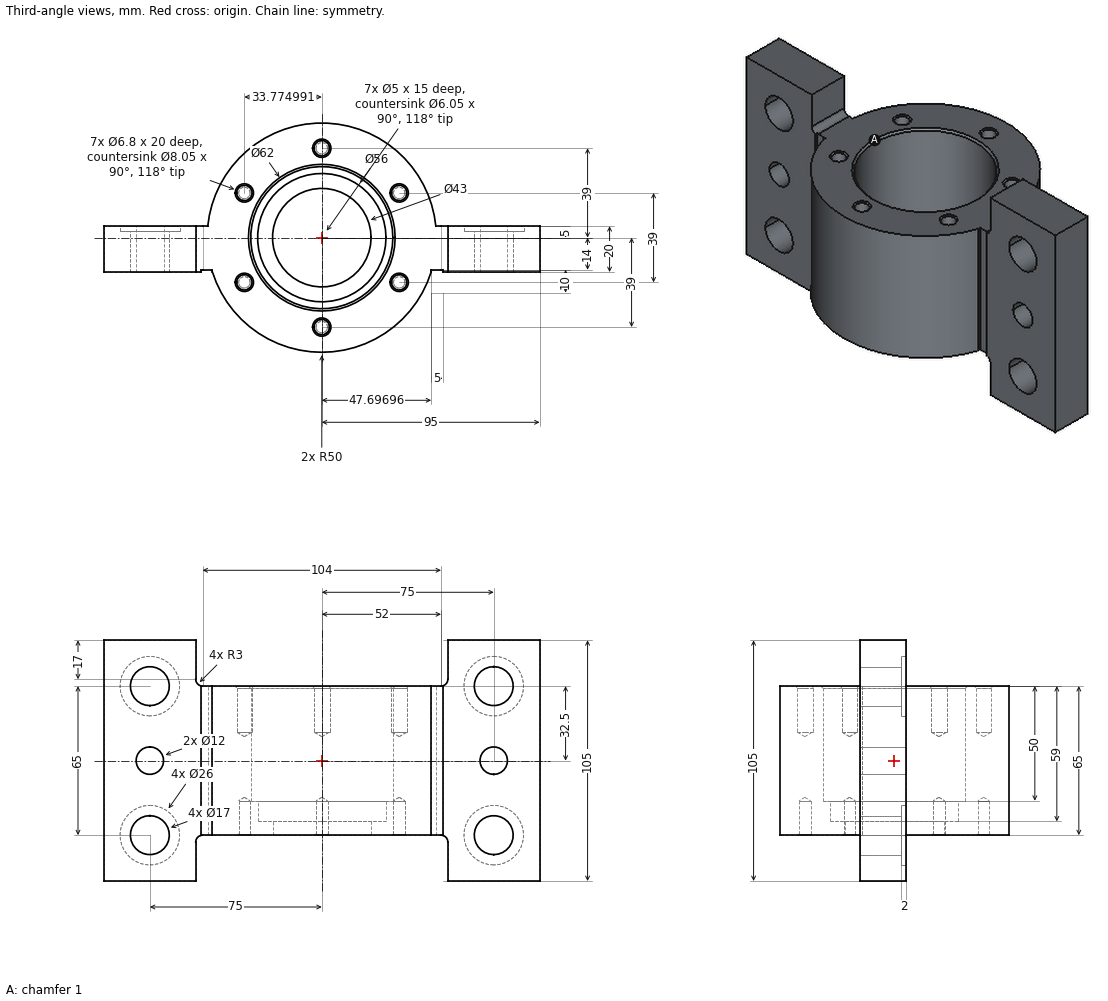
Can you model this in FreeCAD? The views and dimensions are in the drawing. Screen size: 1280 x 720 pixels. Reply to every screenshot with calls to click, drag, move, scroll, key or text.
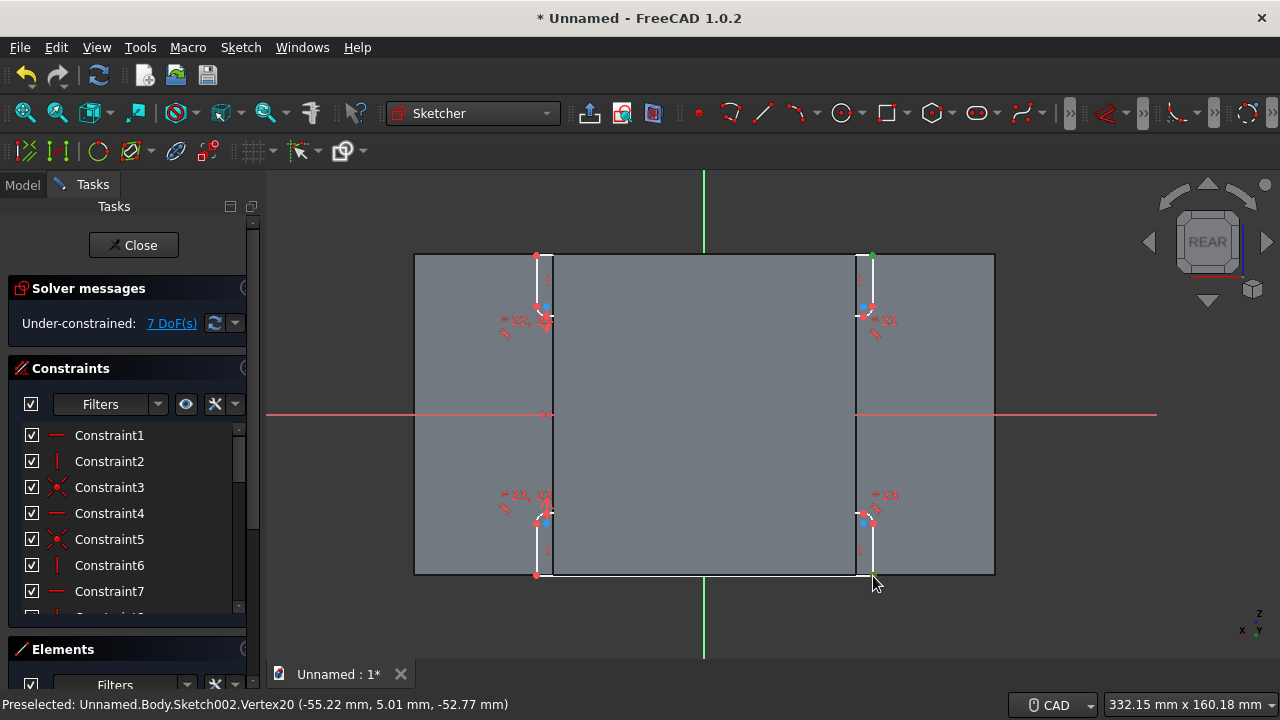
click(353, 415)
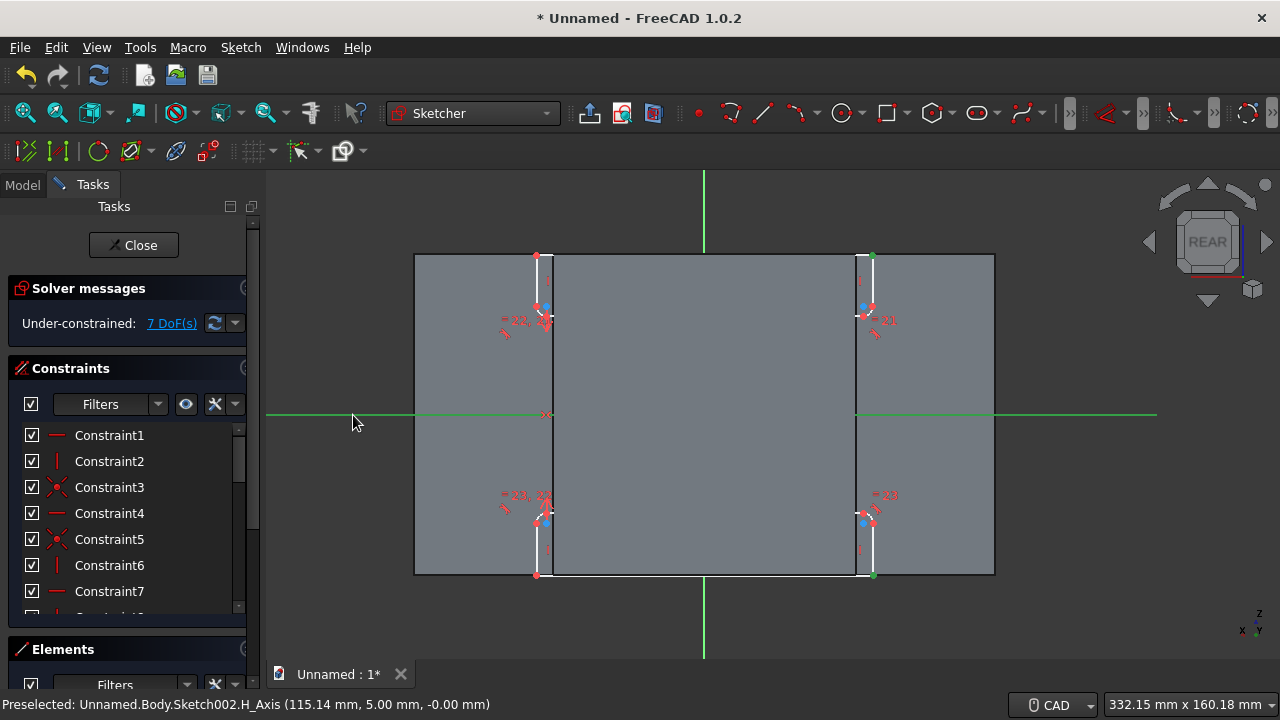
key(s)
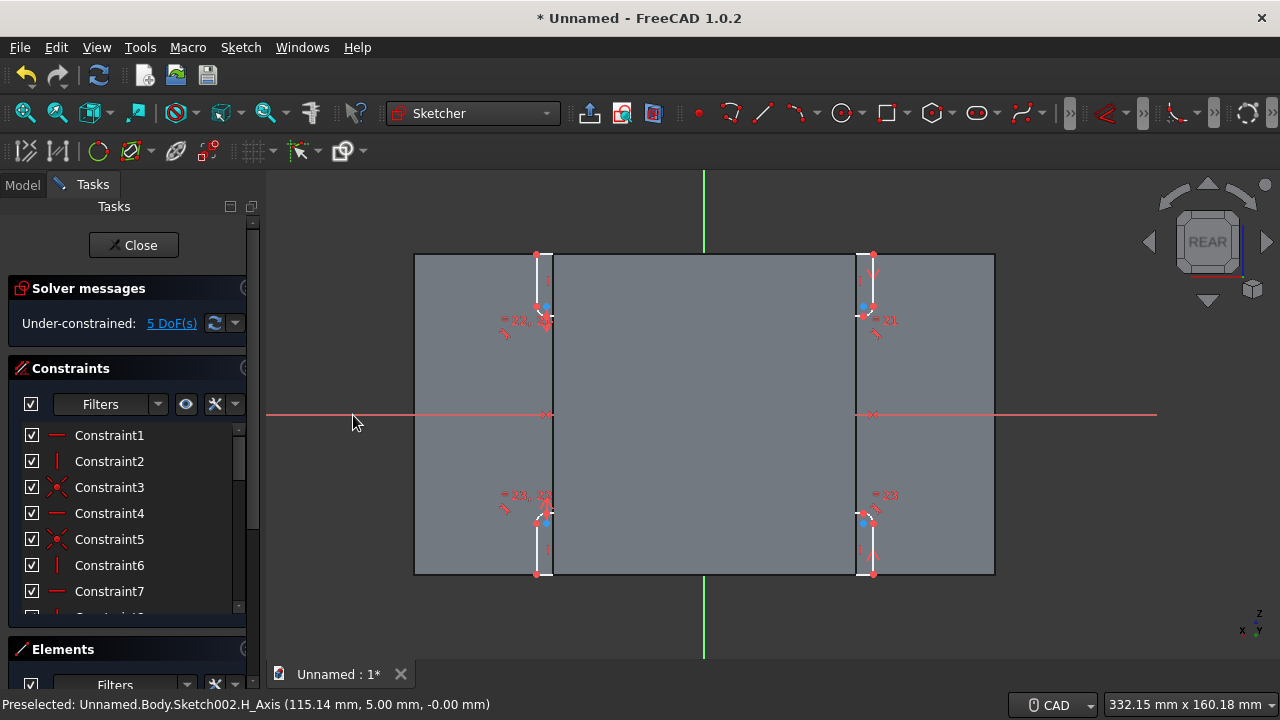
click(1106, 114)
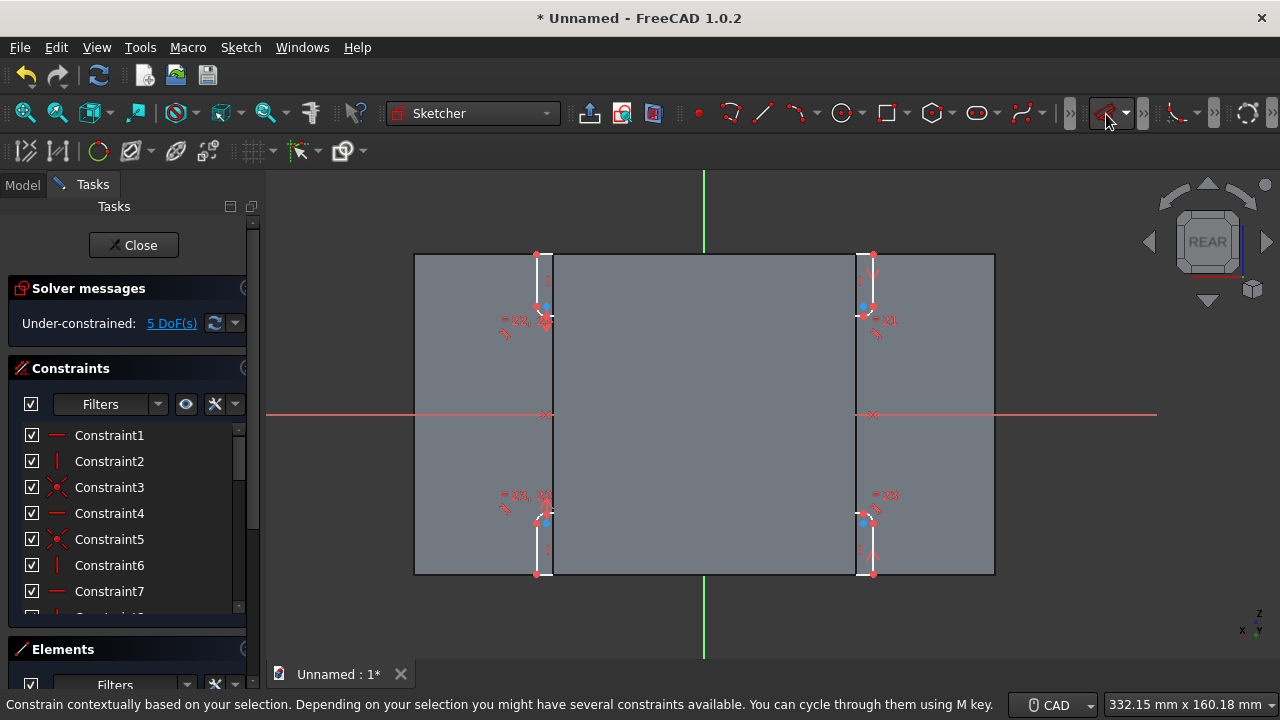
scroll(870, 313, up, 8)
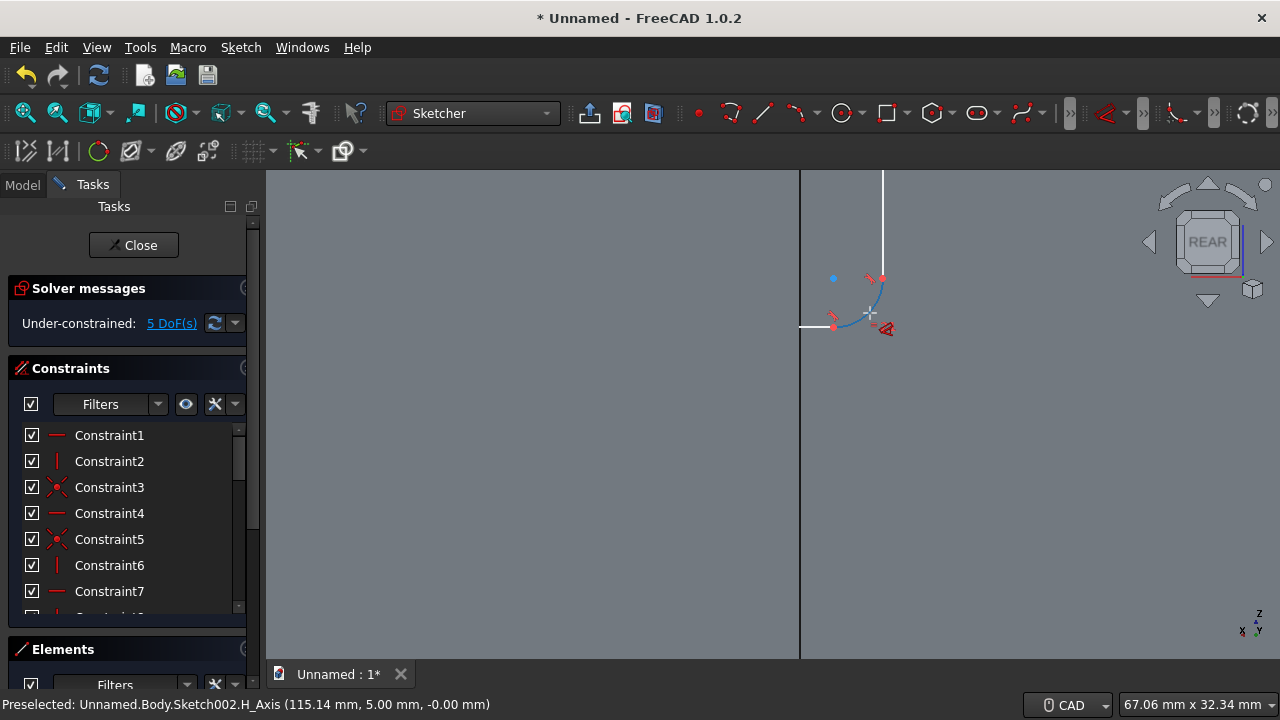
click(869, 313)
click(892, 335)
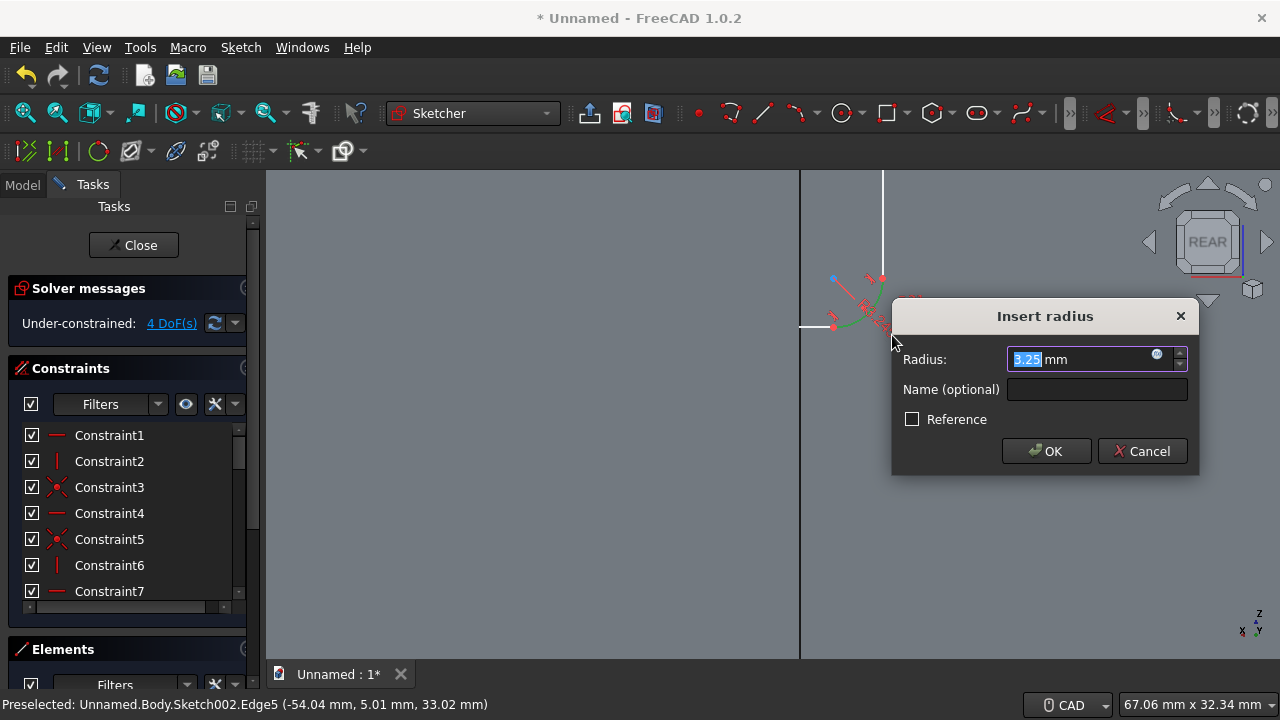
text(3)
key(Return)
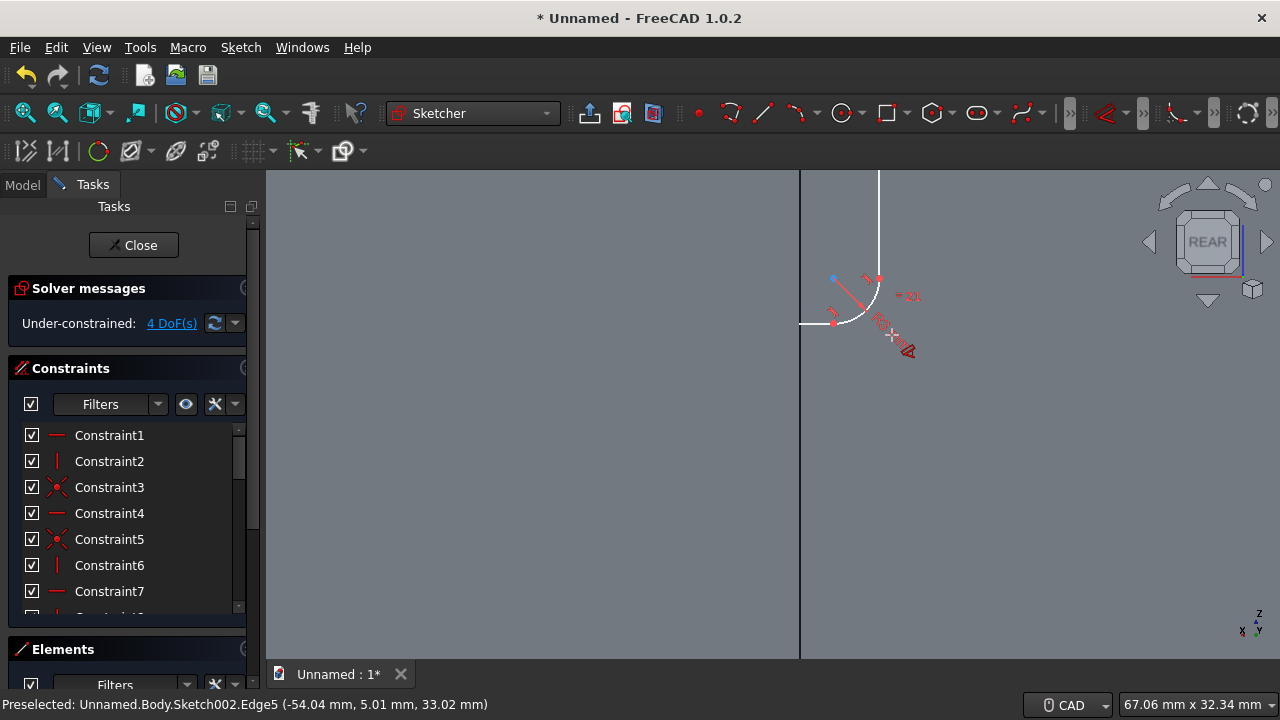
scroll(871, 313, down, 8)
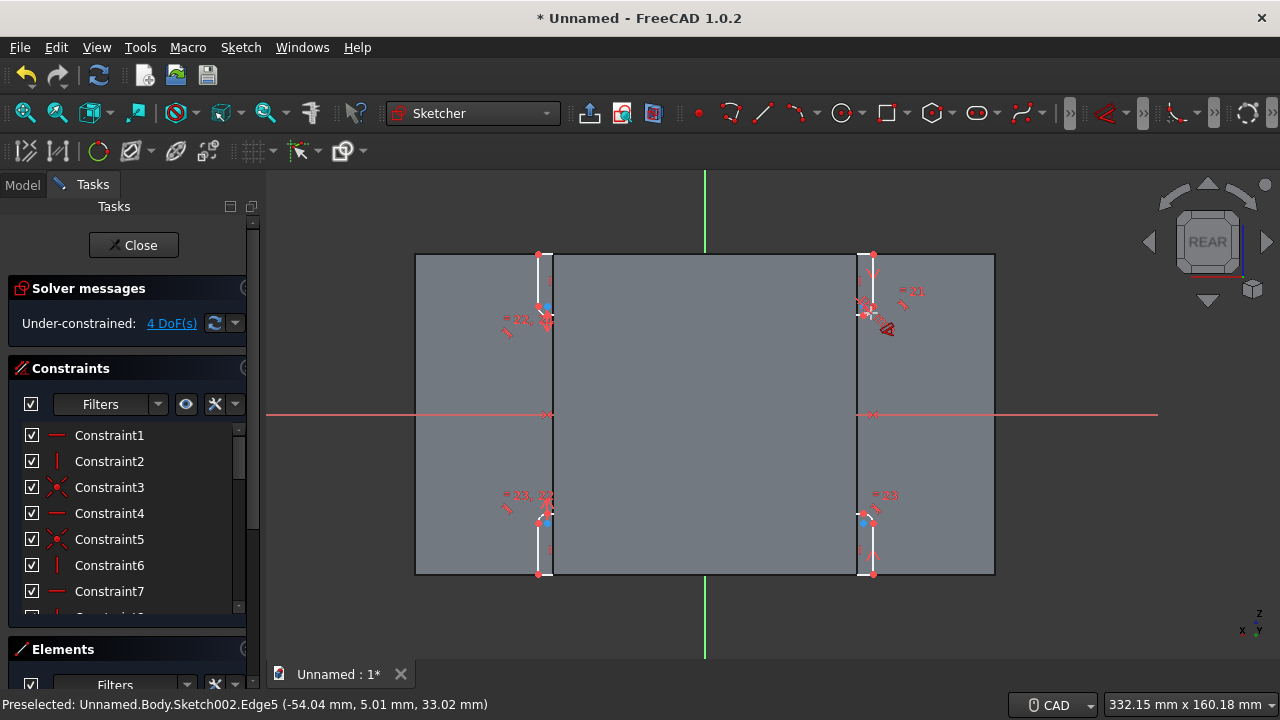
click(873, 291)
click(907, 280)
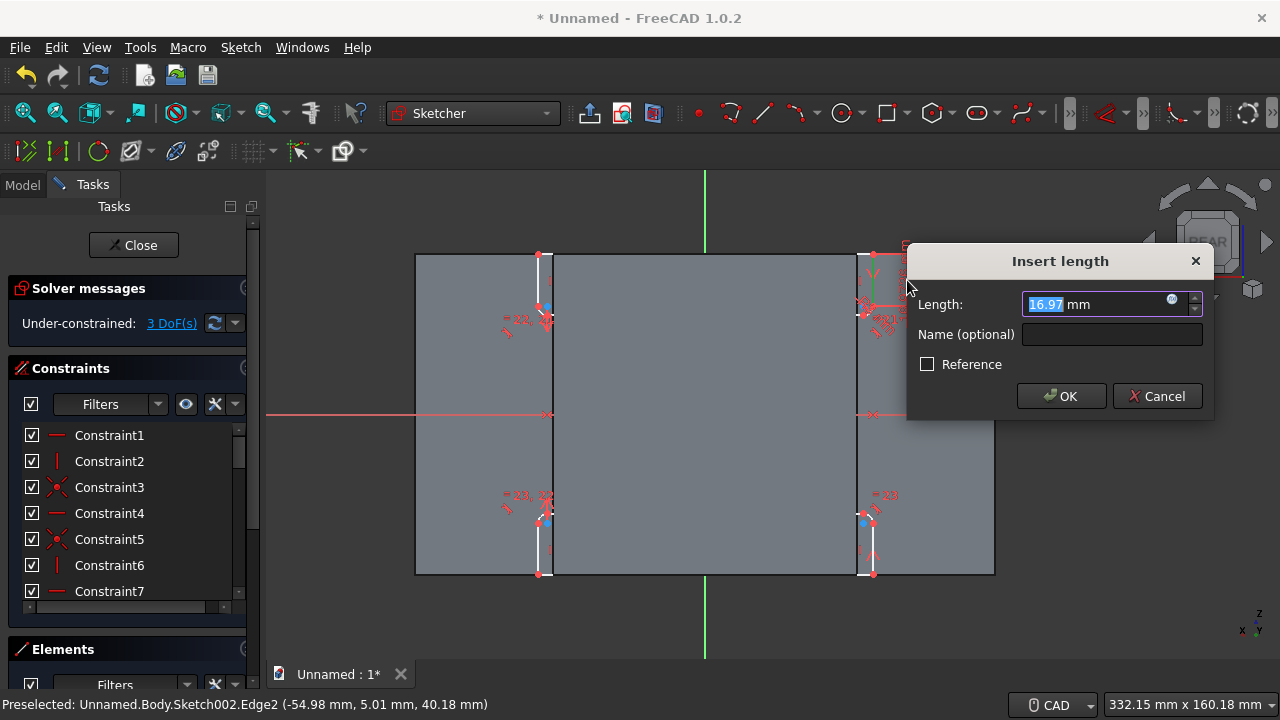
text(17)
key(Return)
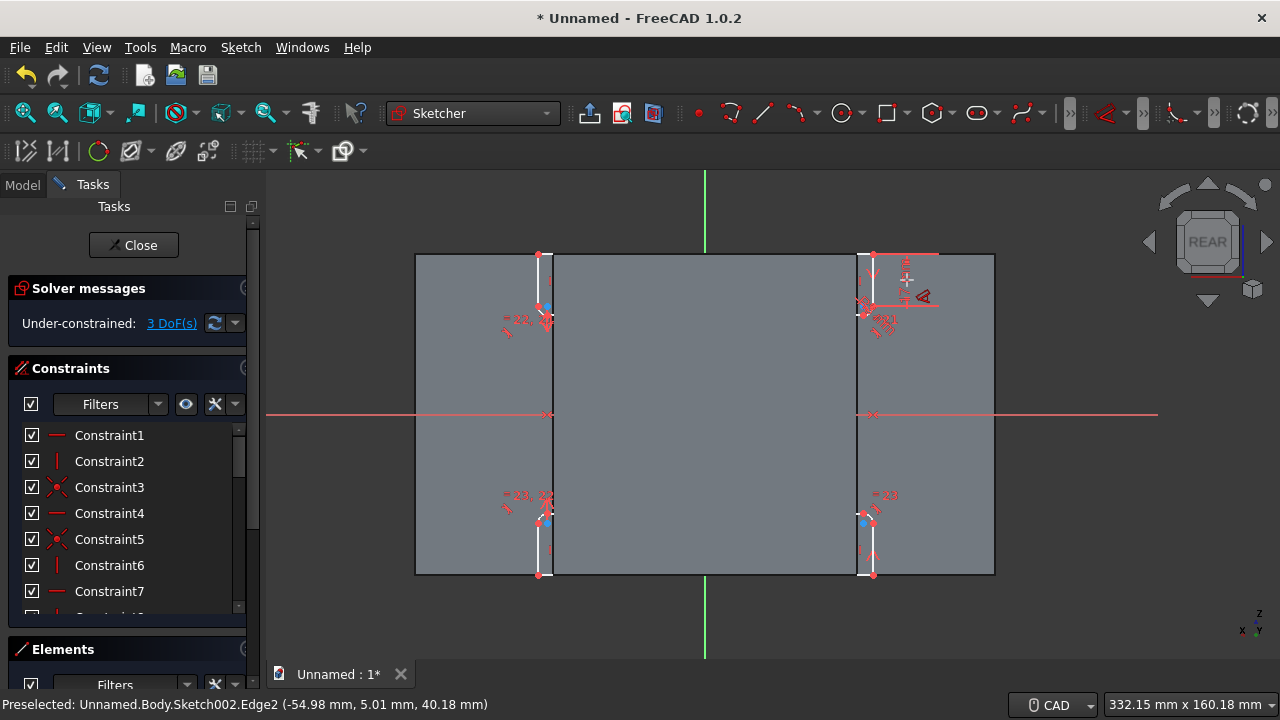
click(642, 315)
click(633, 281)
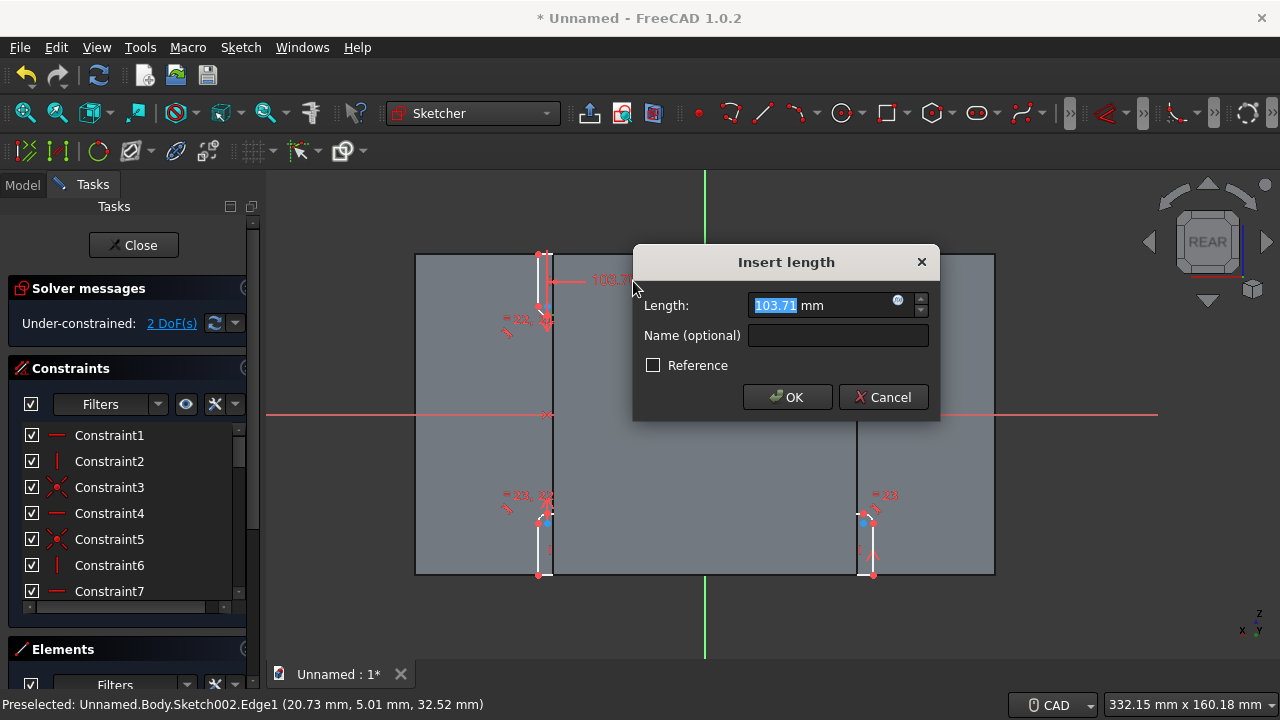
text(104)
key(Return)